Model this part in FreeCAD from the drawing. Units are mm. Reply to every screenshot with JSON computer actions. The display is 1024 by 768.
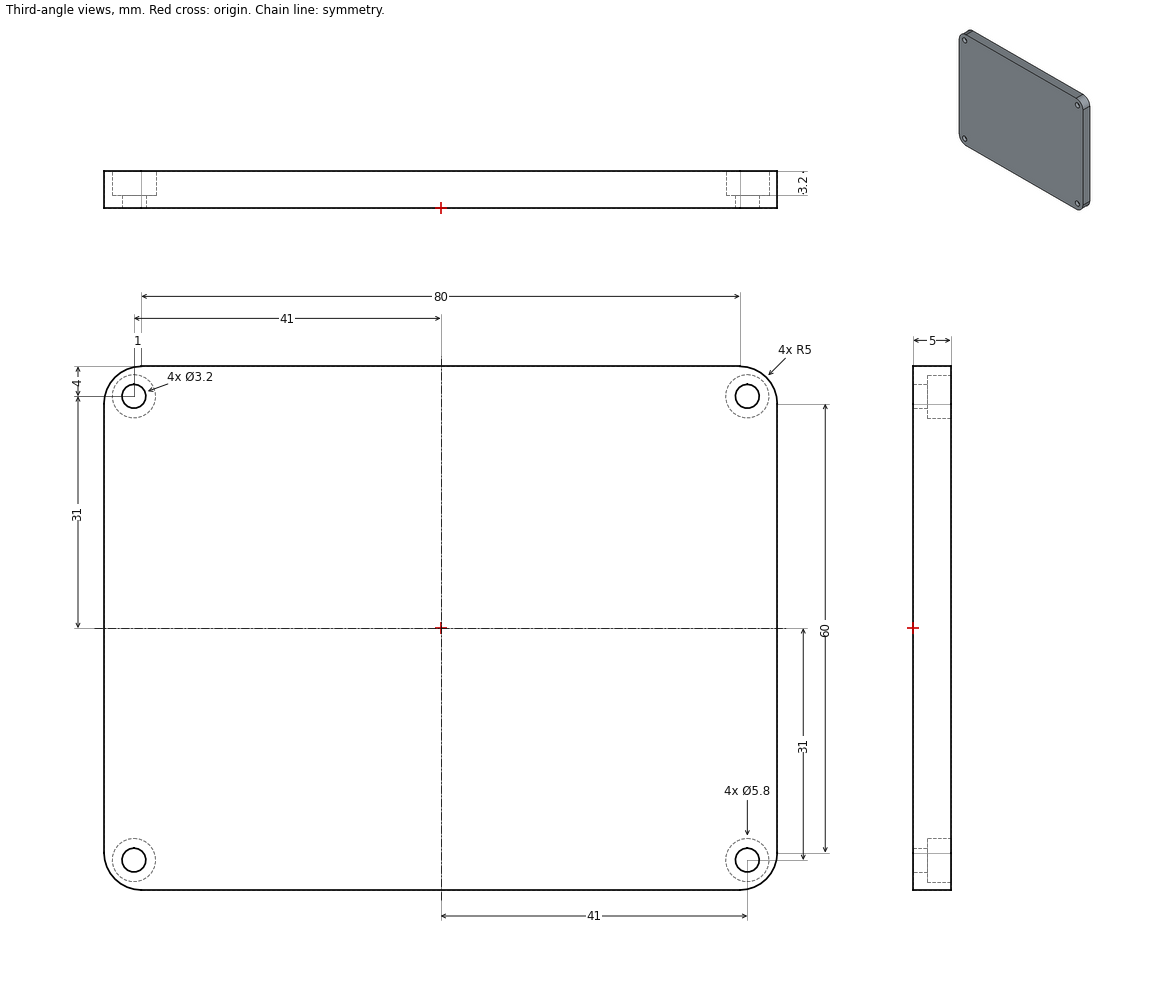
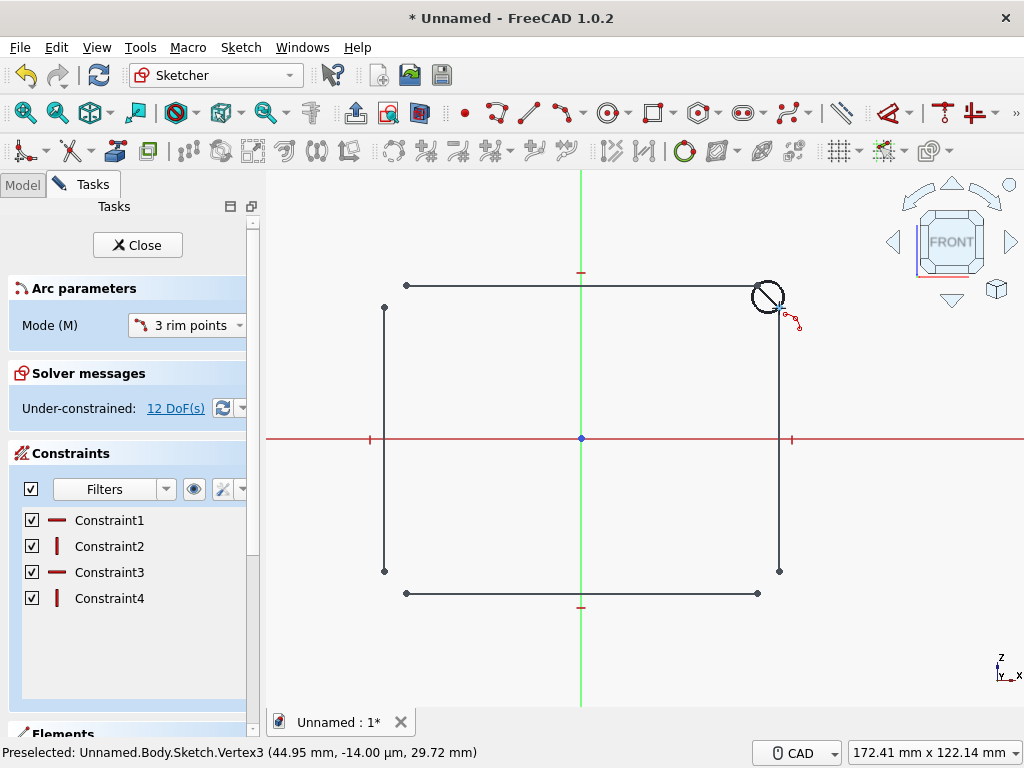
{"action": "scroll", "coordinate": [773, 291], "scroll_direction": "up", "scroll_amount": 5}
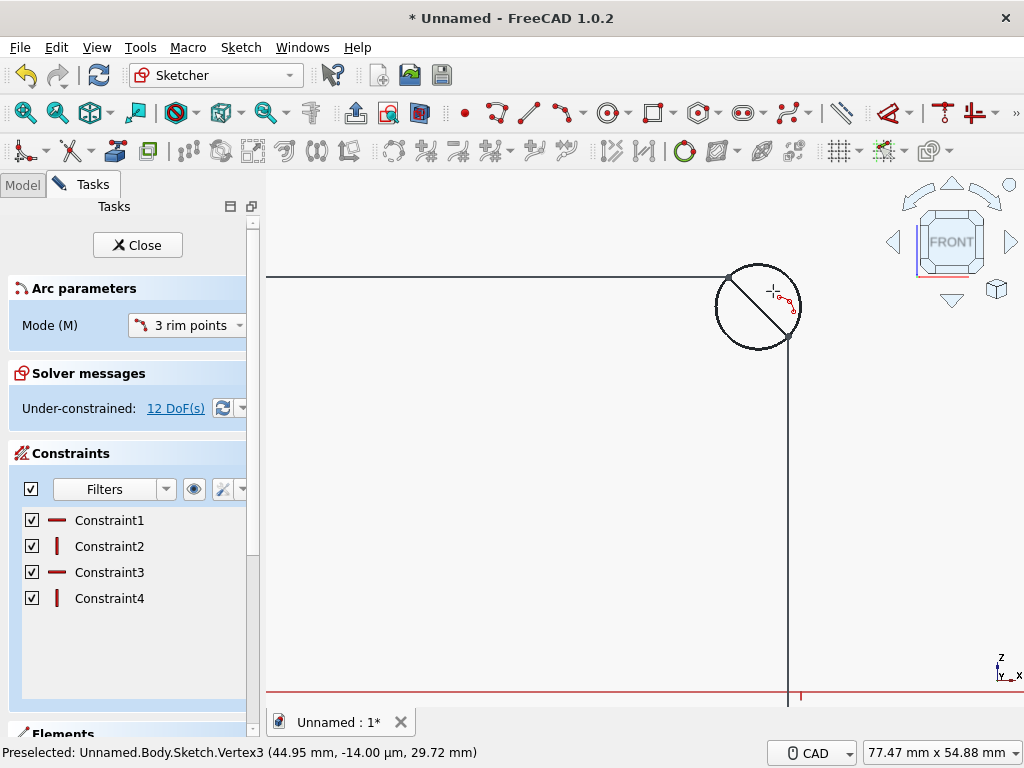
{"action": "left_click", "coordinate": [771, 291]}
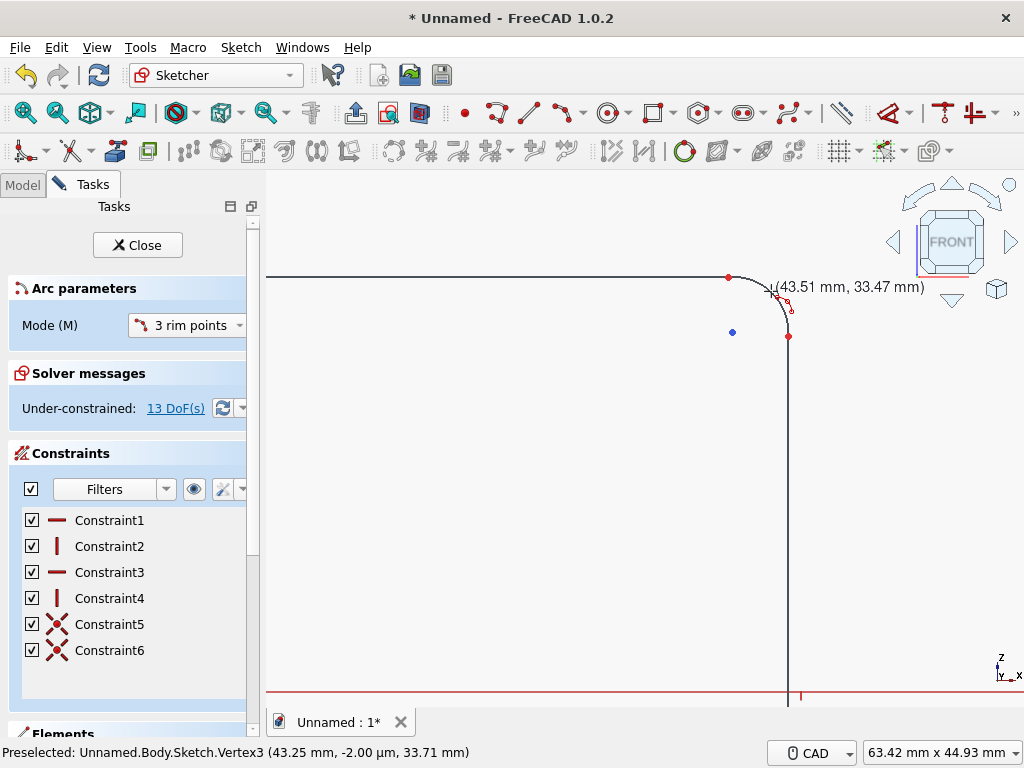
{"action": "scroll", "coordinate": [766, 291], "scroll_direction": "down", "scroll_amount": 5}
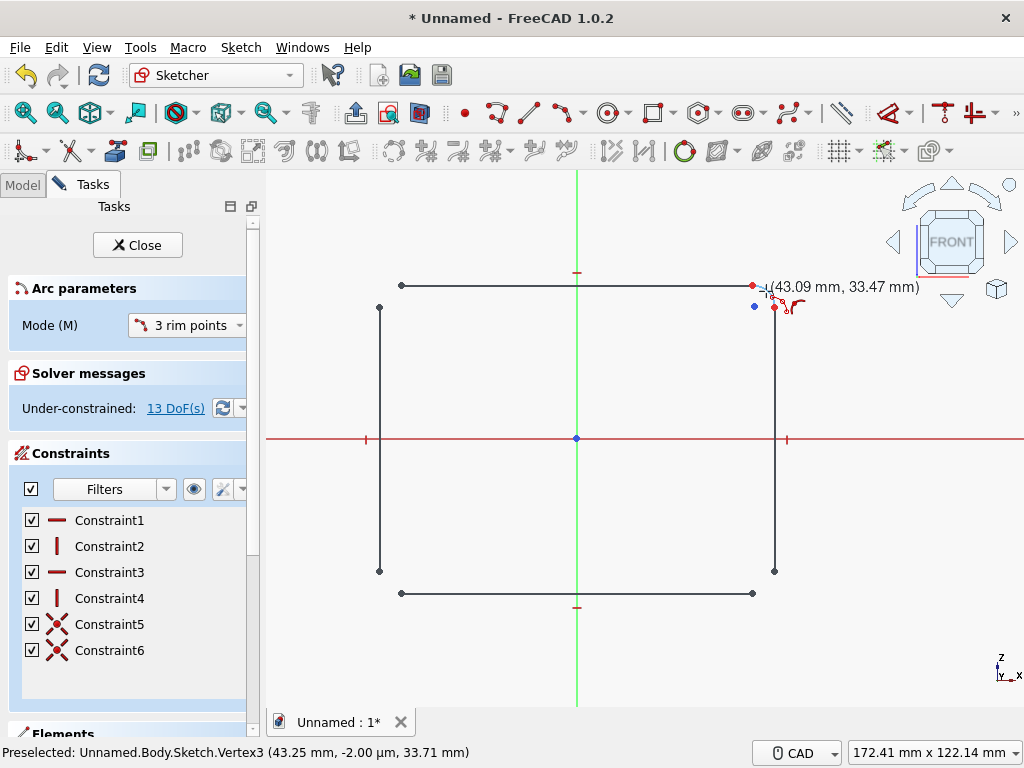
{"action": "left_click", "coordinate": [775, 572]}
{"action": "left_click", "coordinate": [753, 594]}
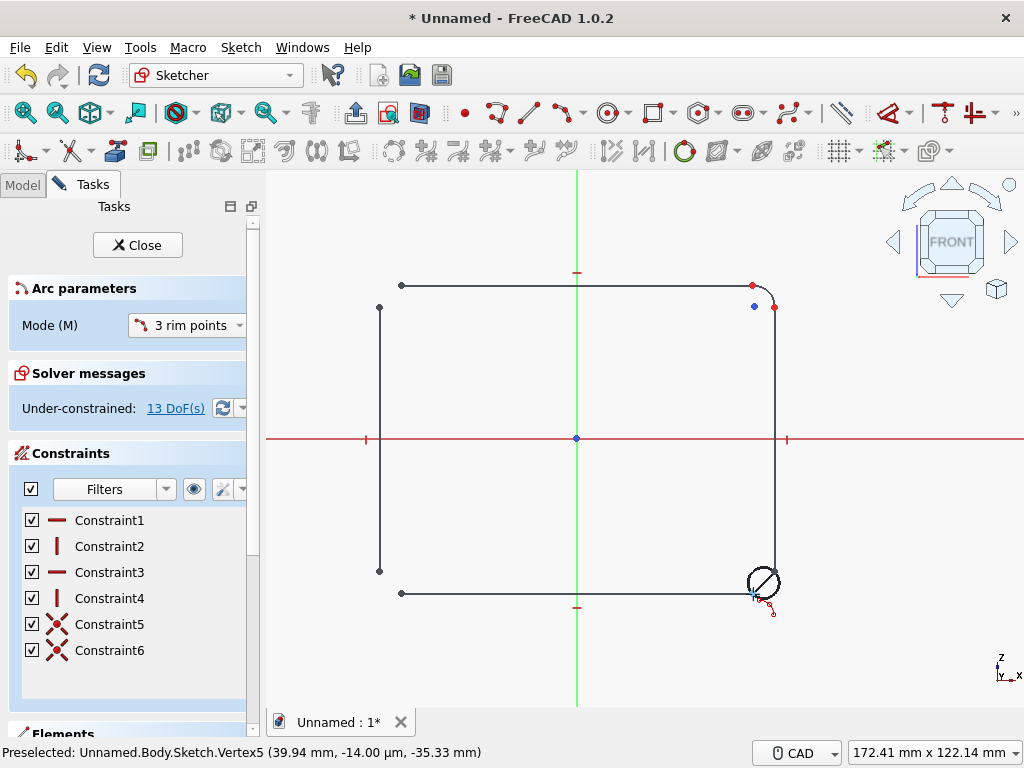
{"action": "scroll", "coordinate": [768, 586], "scroll_direction": "up", "scroll_amount": 5}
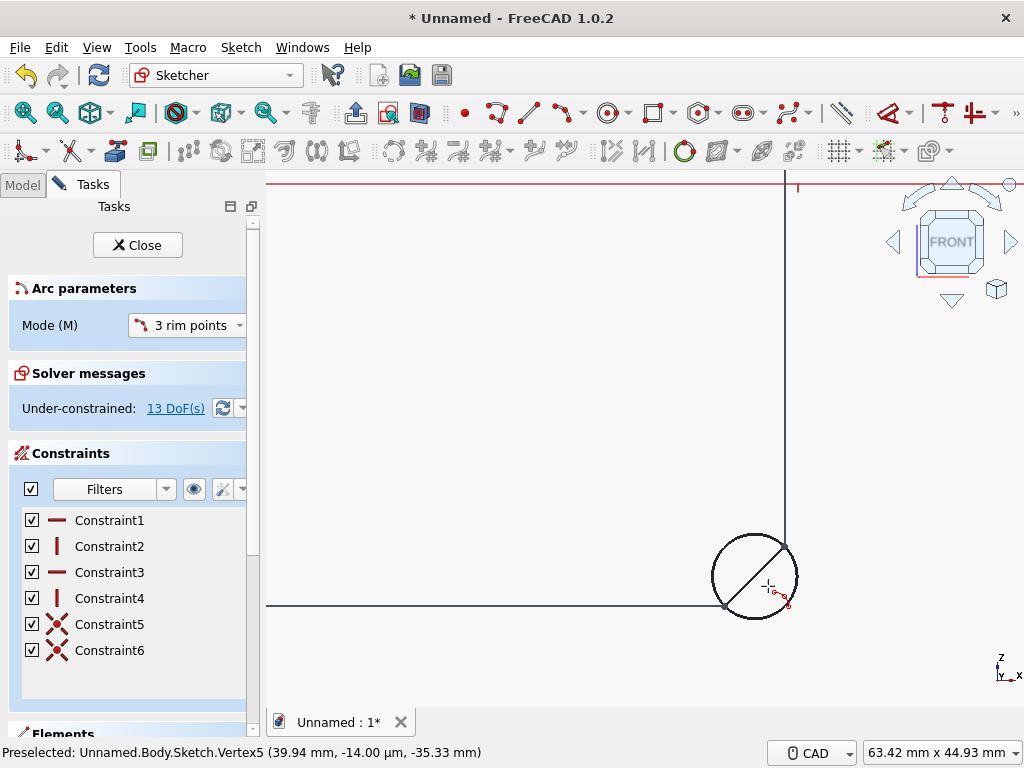
{"action": "left_click", "coordinate": [768, 585]}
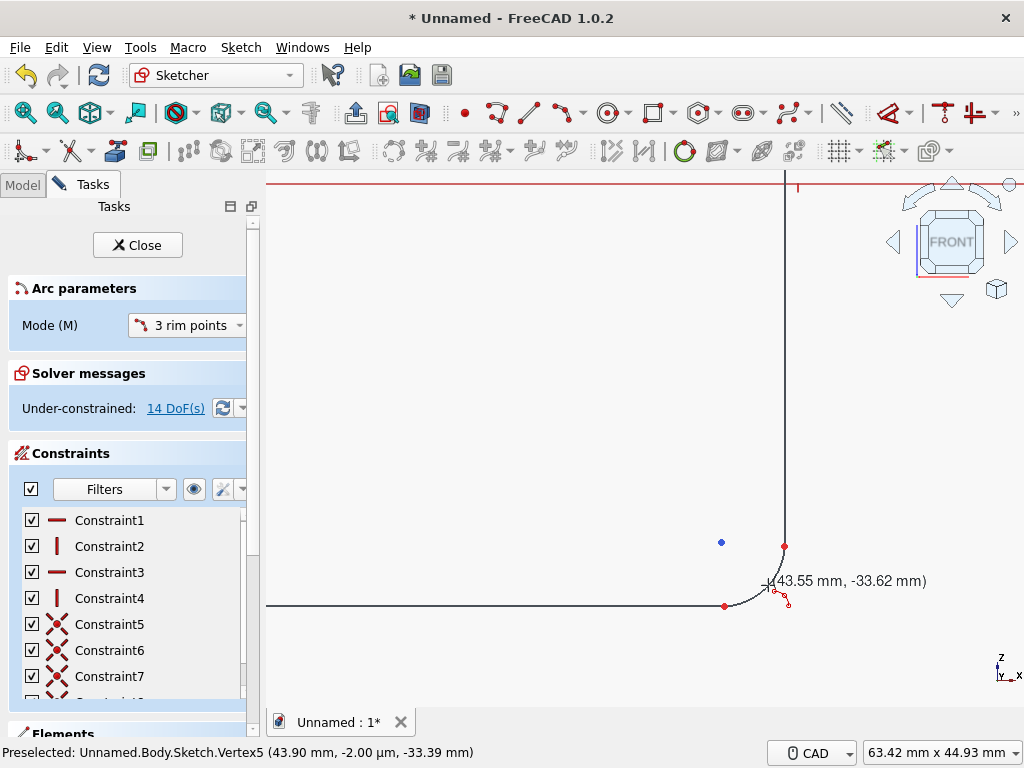
{"action": "scroll", "coordinate": [768, 586], "scroll_direction": "down", "scroll_amount": 5}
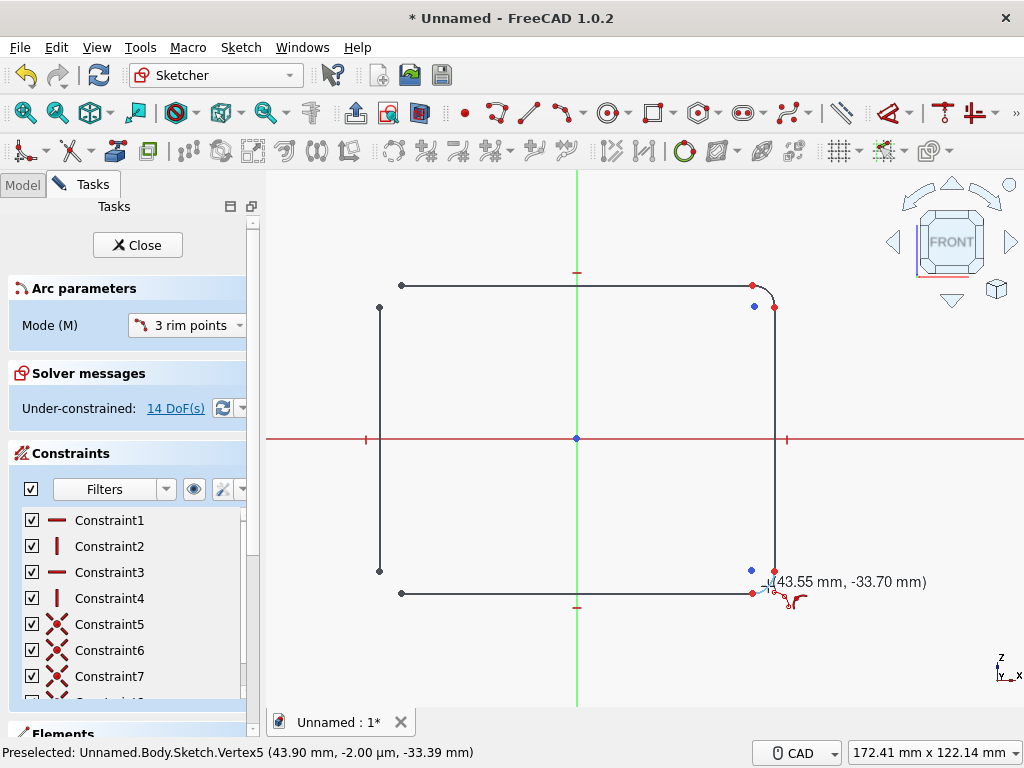
{"action": "left_click", "coordinate": [402, 594]}
{"action": "left_click", "coordinate": [380, 572]}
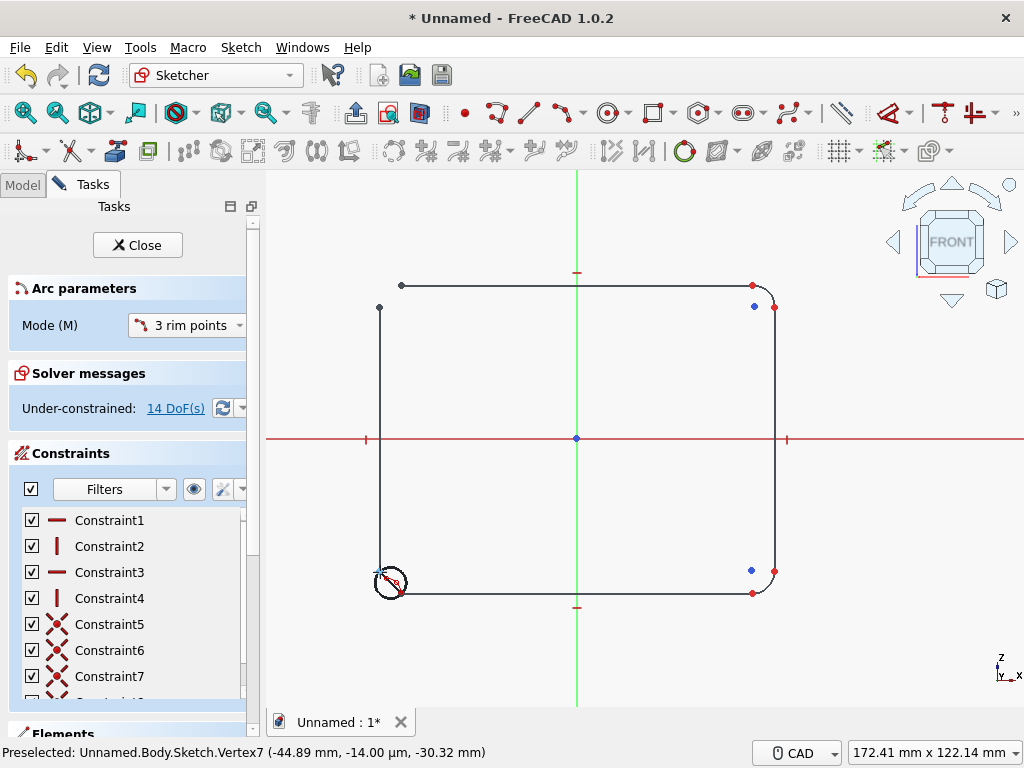
{"action": "scroll", "coordinate": [386, 586], "scroll_direction": "up", "scroll_amount": 5}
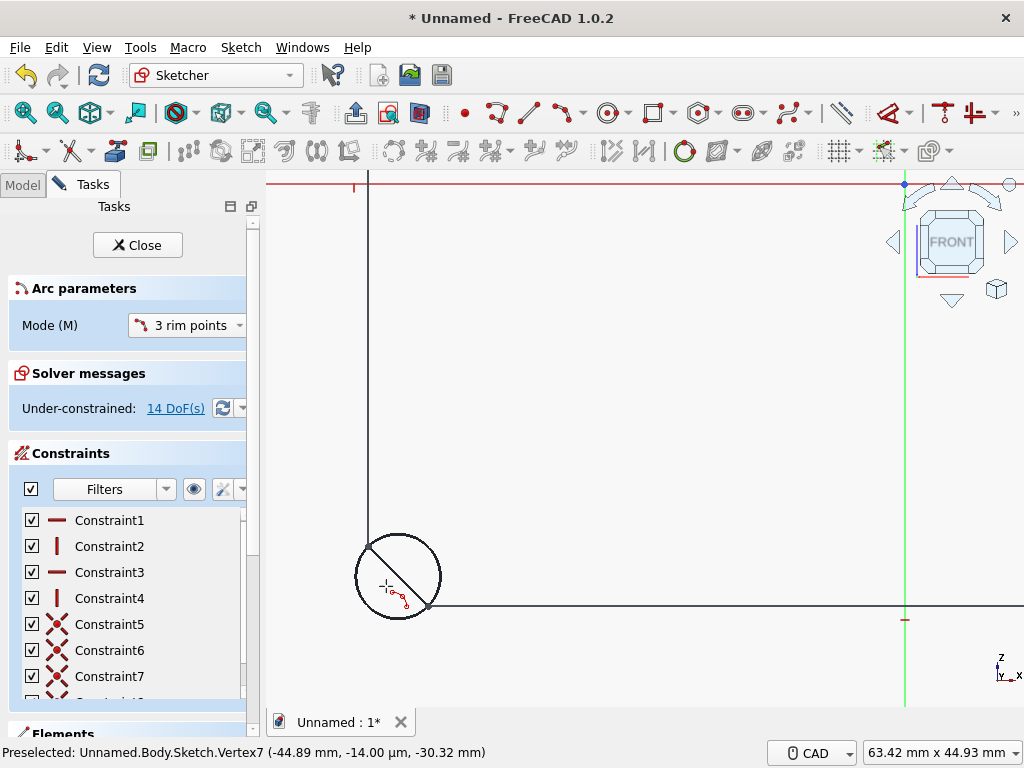
{"action": "left_click", "coordinate": [384, 585]}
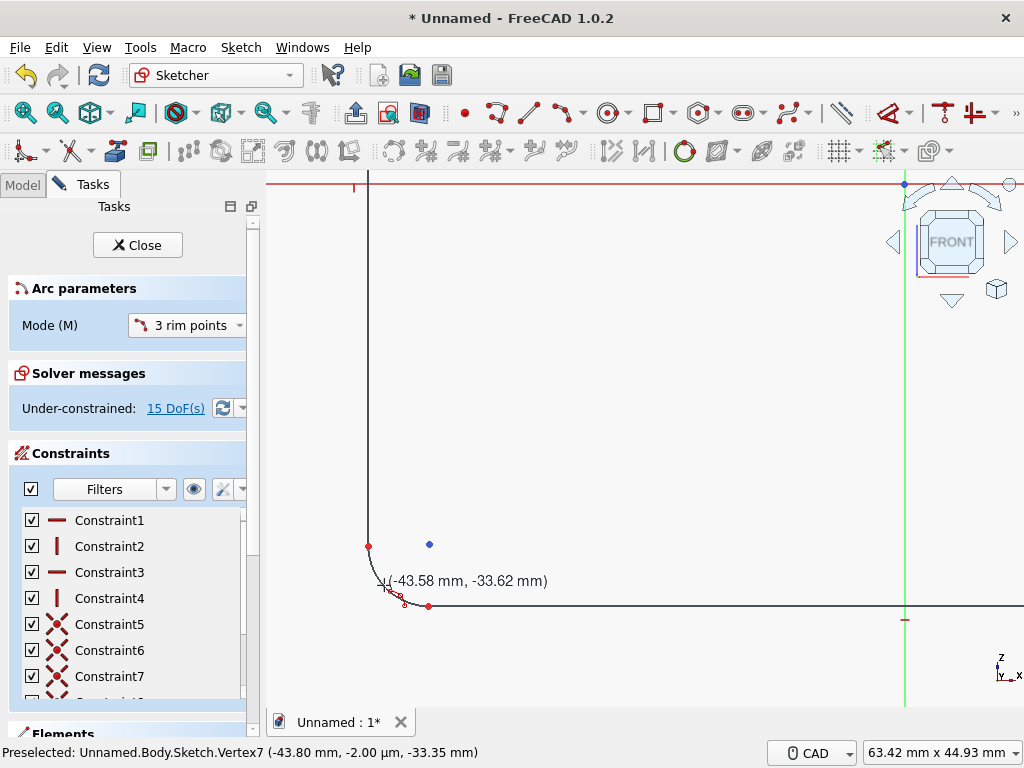
{"action": "scroll", "coordinate": [385, 586], "scroll_direction": "down", "scroll_amount": 5}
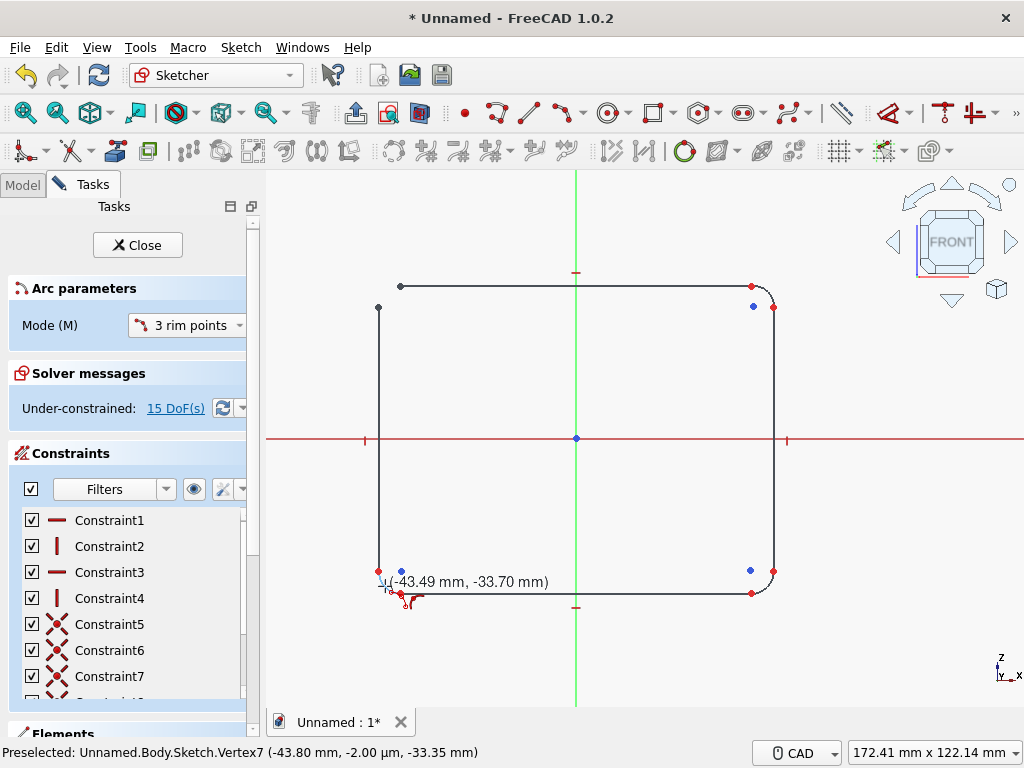
{"action": "left_click", "coordinate": [379, 308]}
{"action": "left_click", "coordinate": [401, 286]}